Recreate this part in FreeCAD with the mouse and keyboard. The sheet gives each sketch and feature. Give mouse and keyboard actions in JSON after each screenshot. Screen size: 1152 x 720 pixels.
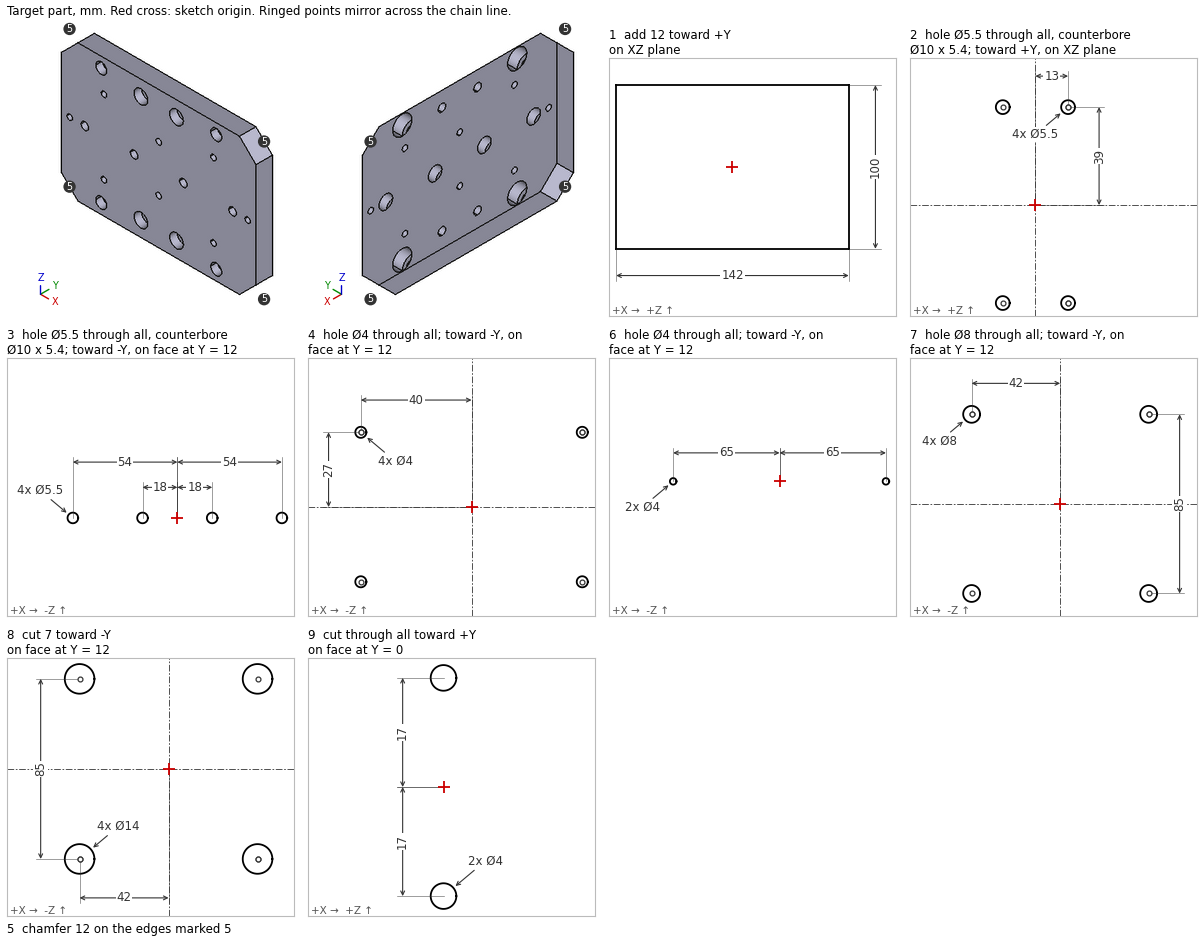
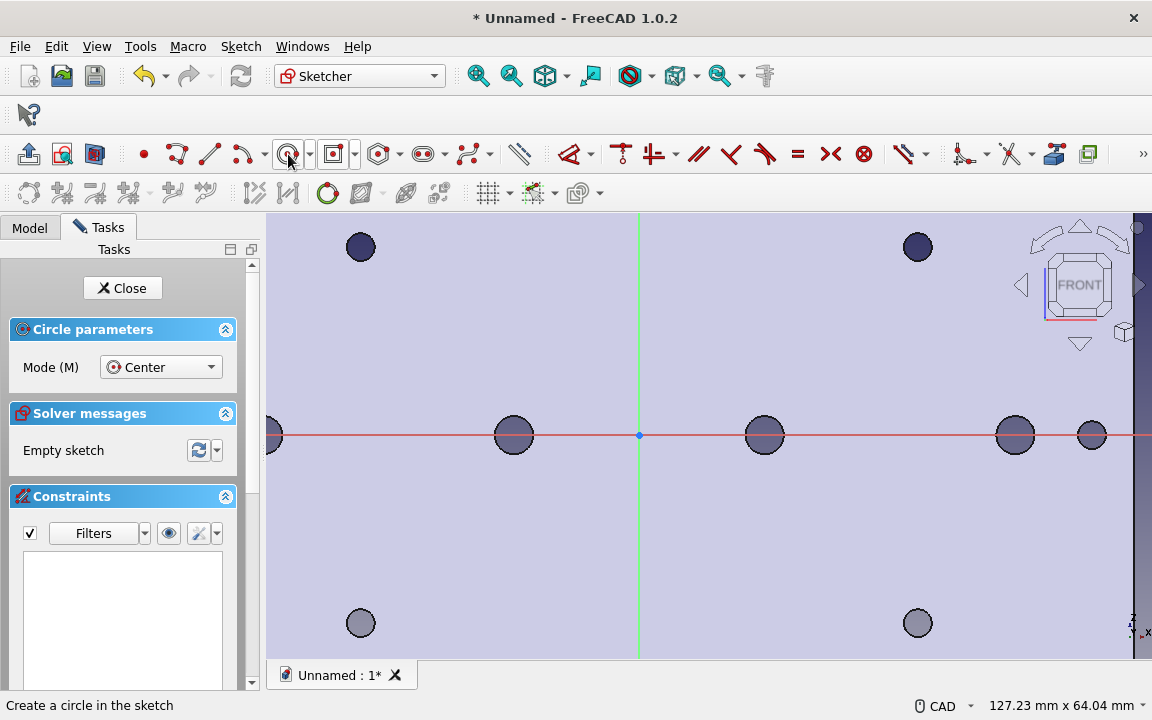
{"action": "scroll", "coordinate": [639, 554], "scroll_direction": "up", "scroll_amount": 3}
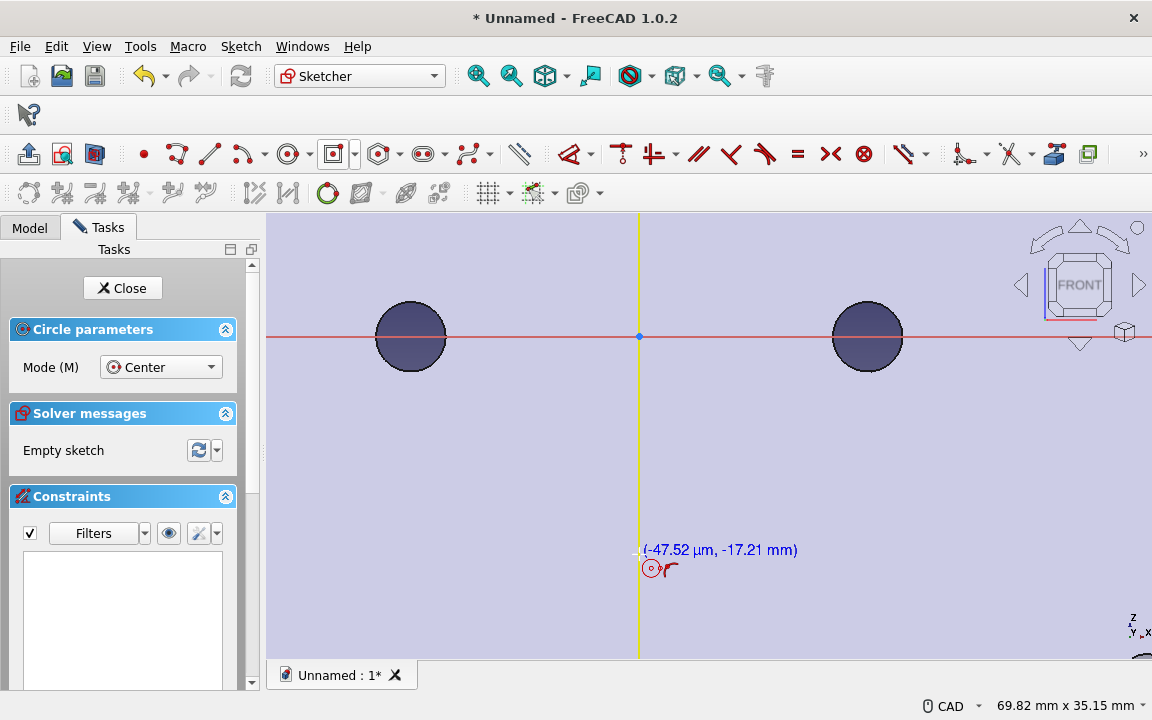
{"action": "left_click", "coordinate": [639, 553]}
{"action": "left_click", "coordinate": [657, 535]}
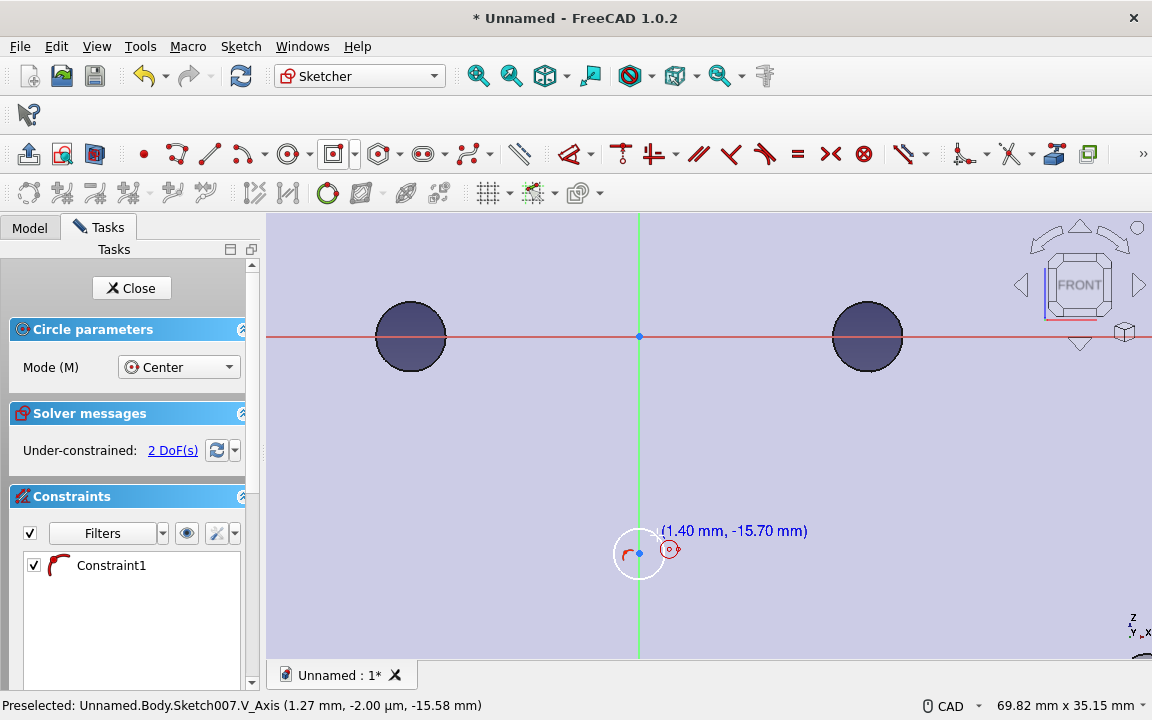
{"action": "scroll", "coordinate": [642, 557], "scroll_direction": "down", "scroll_amount": 3}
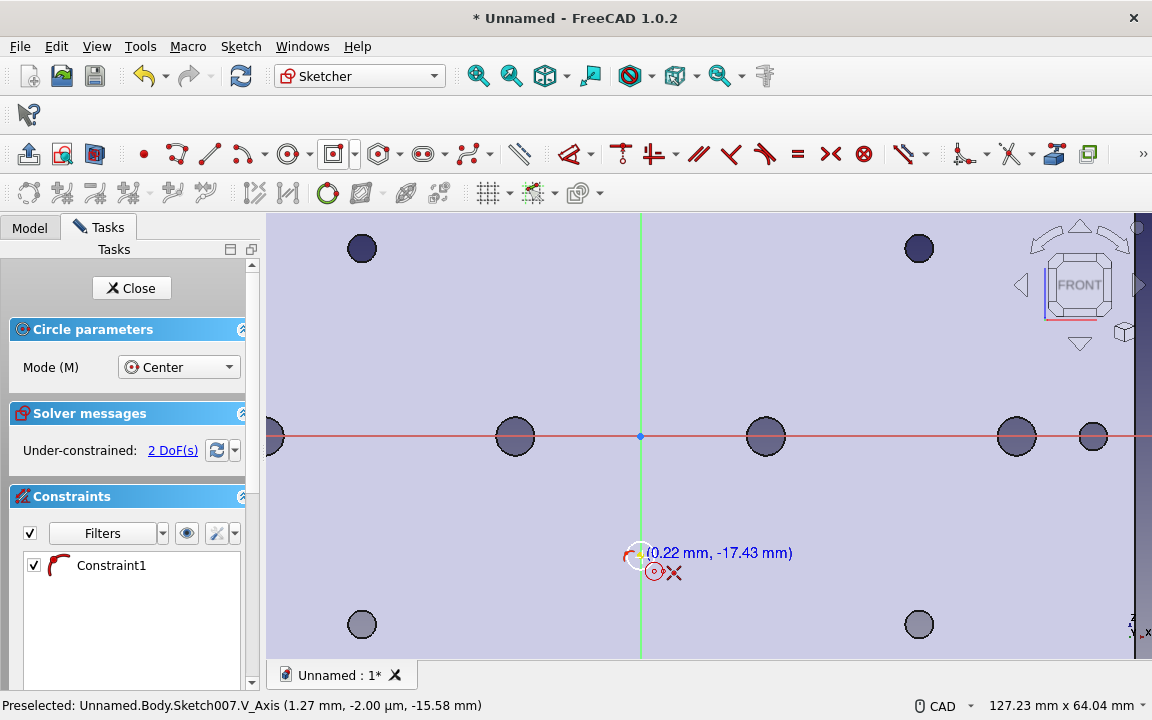
{"action": "scroll", "coordinate": [641, 318], "scroll_direction": "up", "scroll_amount": 3}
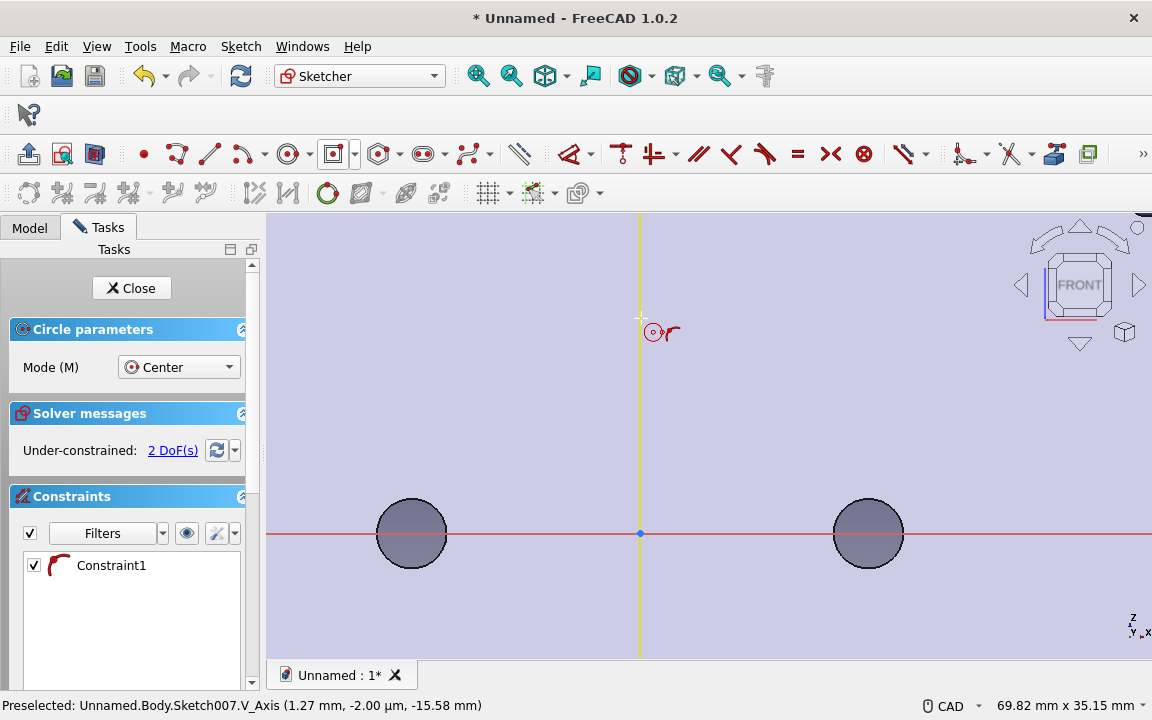
{"action": "left_click", "coordinate": [640, 318]}
{"action": "left_click", "coordinate": [658, 300]}
{"action": "key", "text": "Escape"}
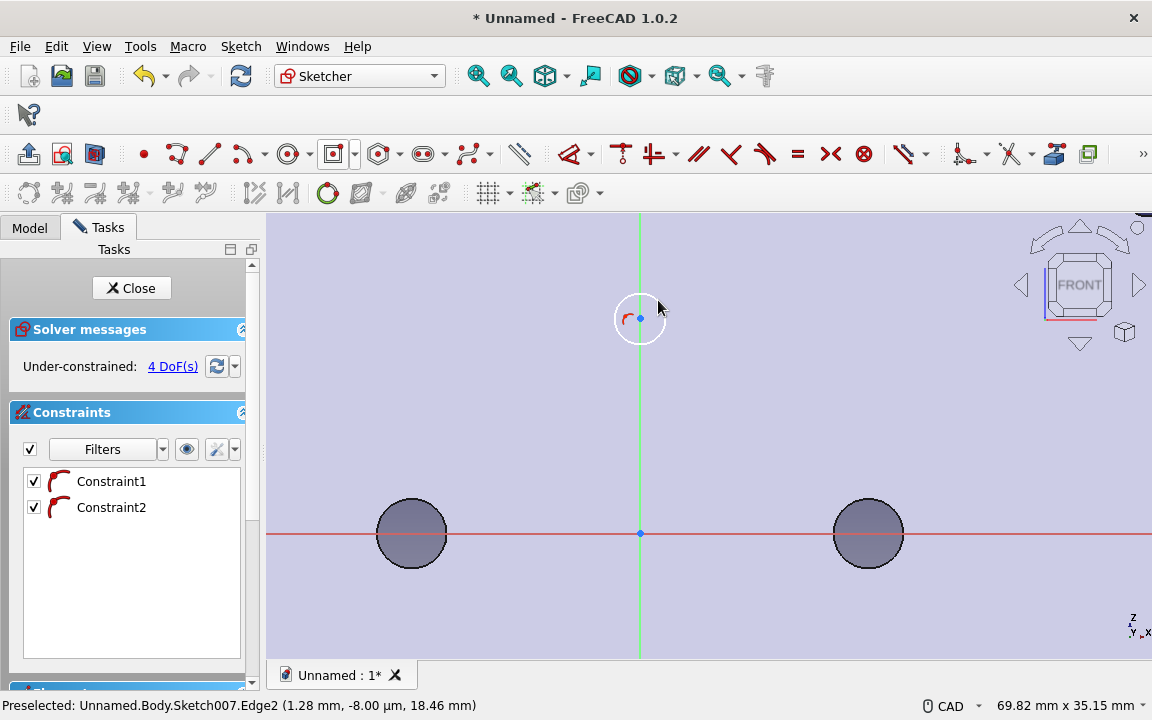
{"action": "scroll", "coordinate": [641, 317], "scroll_direction": "down", "scroll_amount": 3}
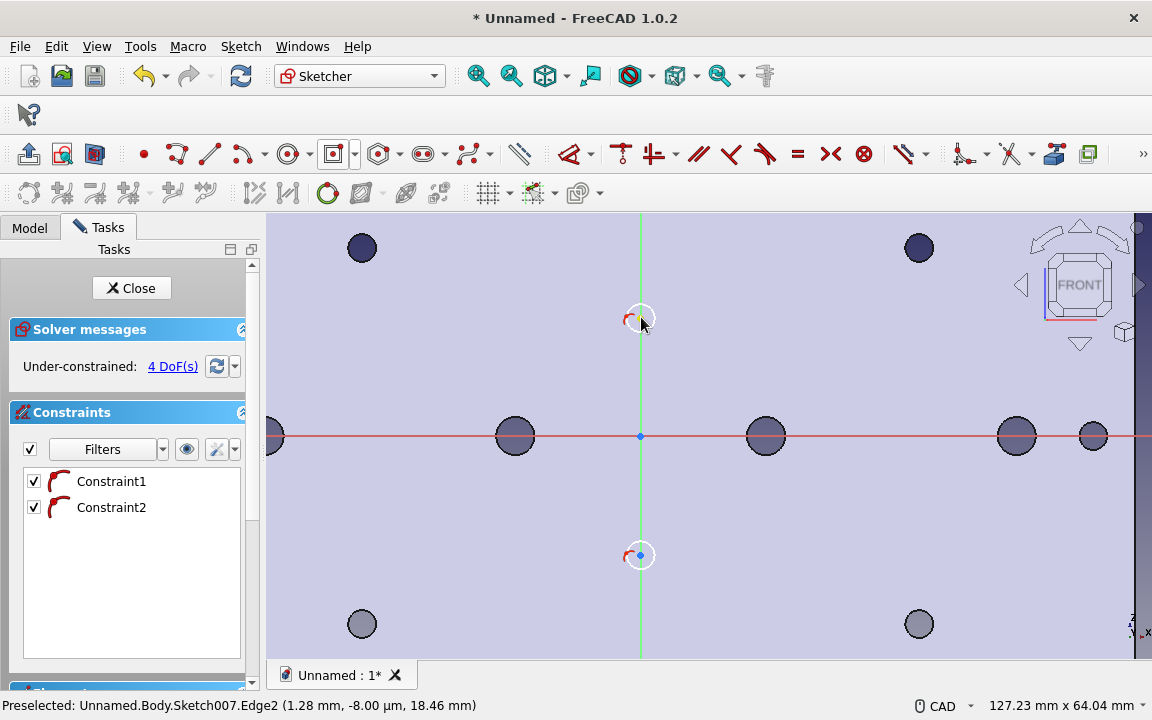
{"action": "scroll", "coordinate": [650, 545], "scroll_direction": "up", "scroll_amount": 2}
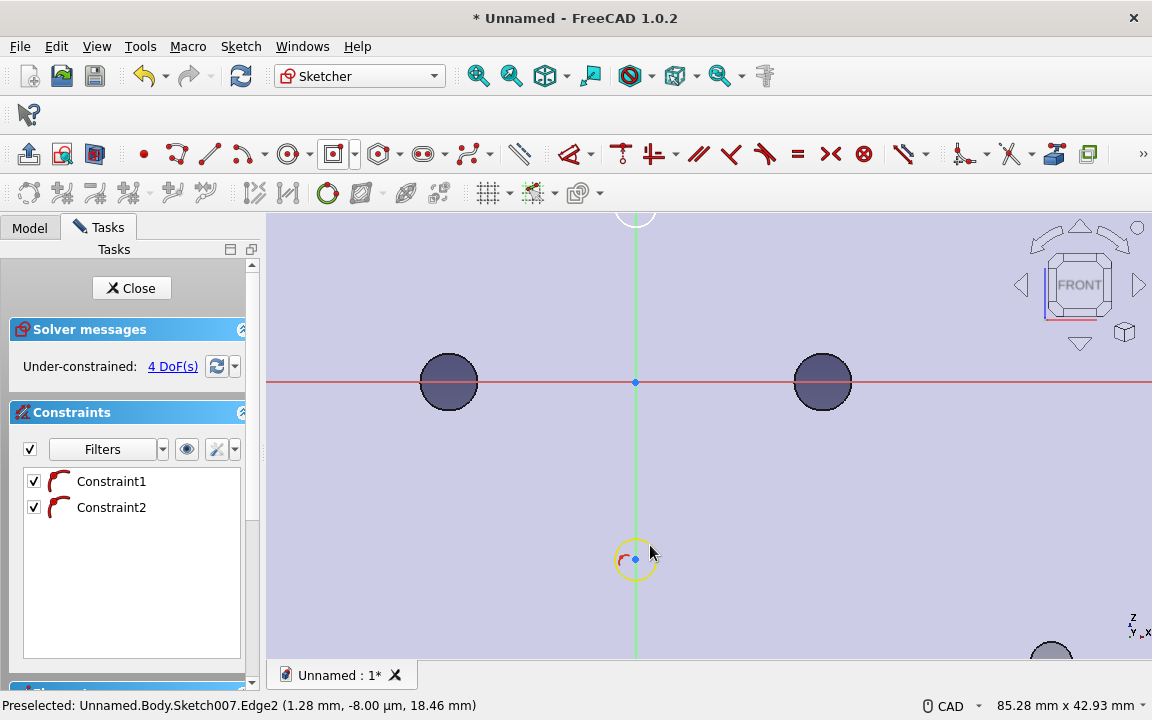
{"action": "left_click", "coordinate": [650, 545]}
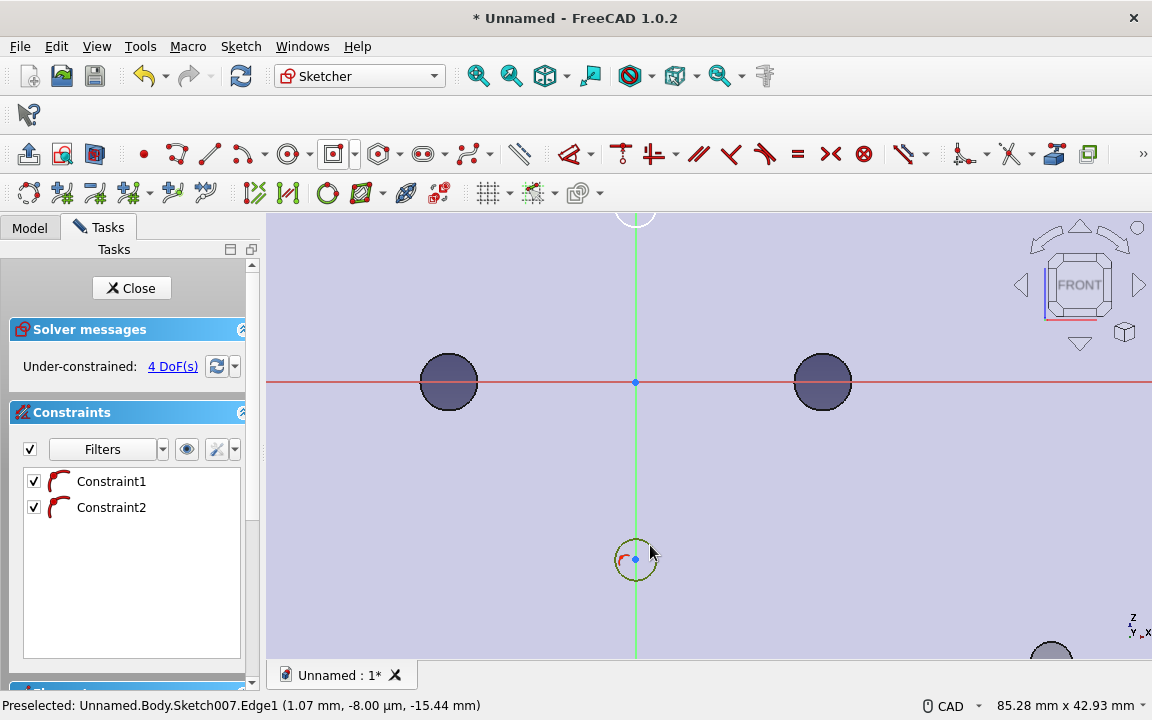
{"action": "scroll", "coordinate": [650, 546], "scroll_direction": "down", "scroll_amount": 2}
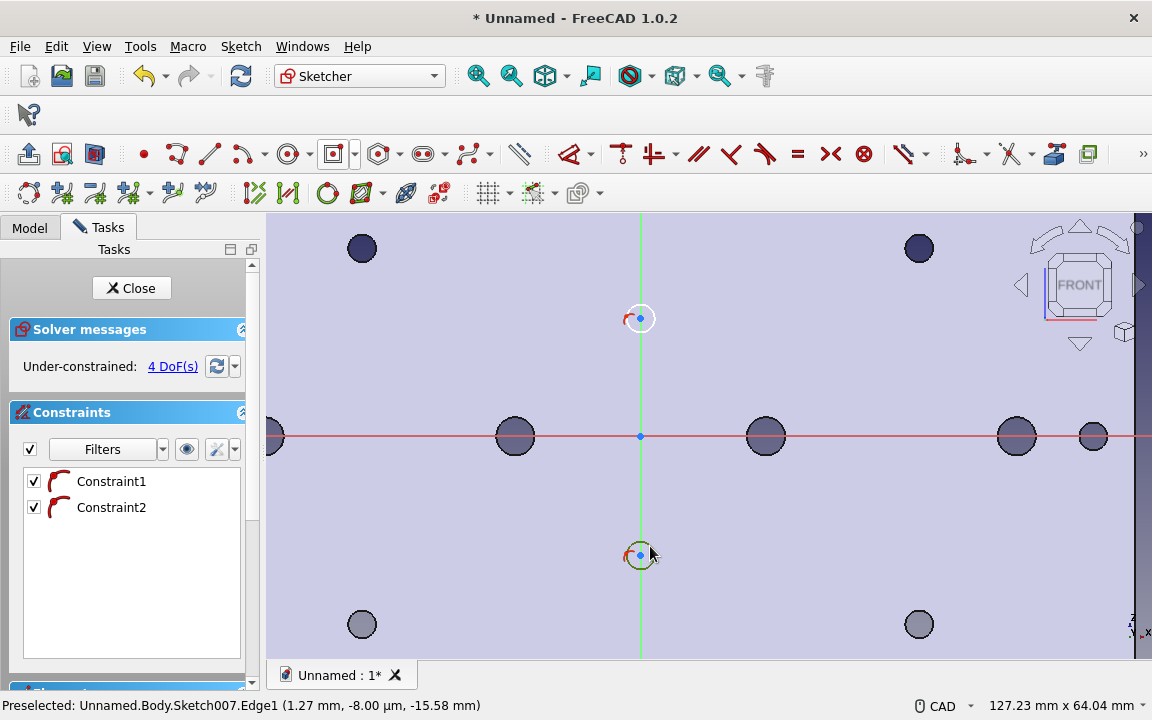
{"action": "scroll", "coordinate": [651, 309], "scroll_direction": "up", "scroll_amount": 2}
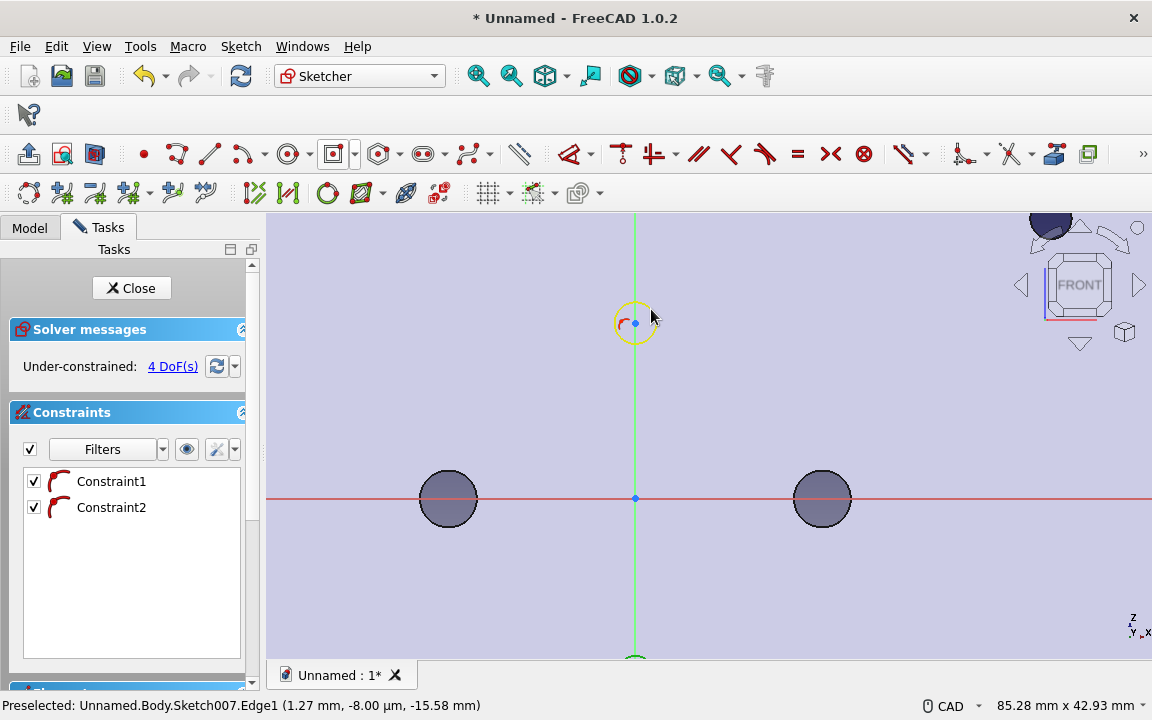
{"action": "left_click", "coordinate": [650, 308]}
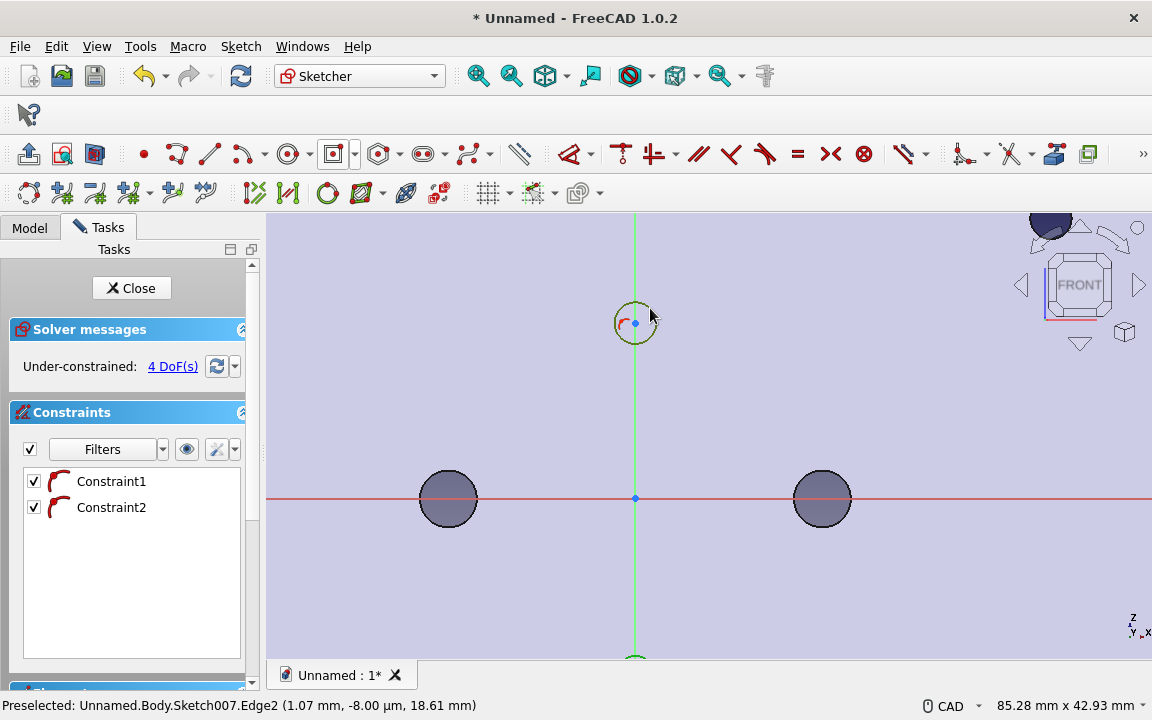
{"action": "left_click", "coordinate": [798, 154]}